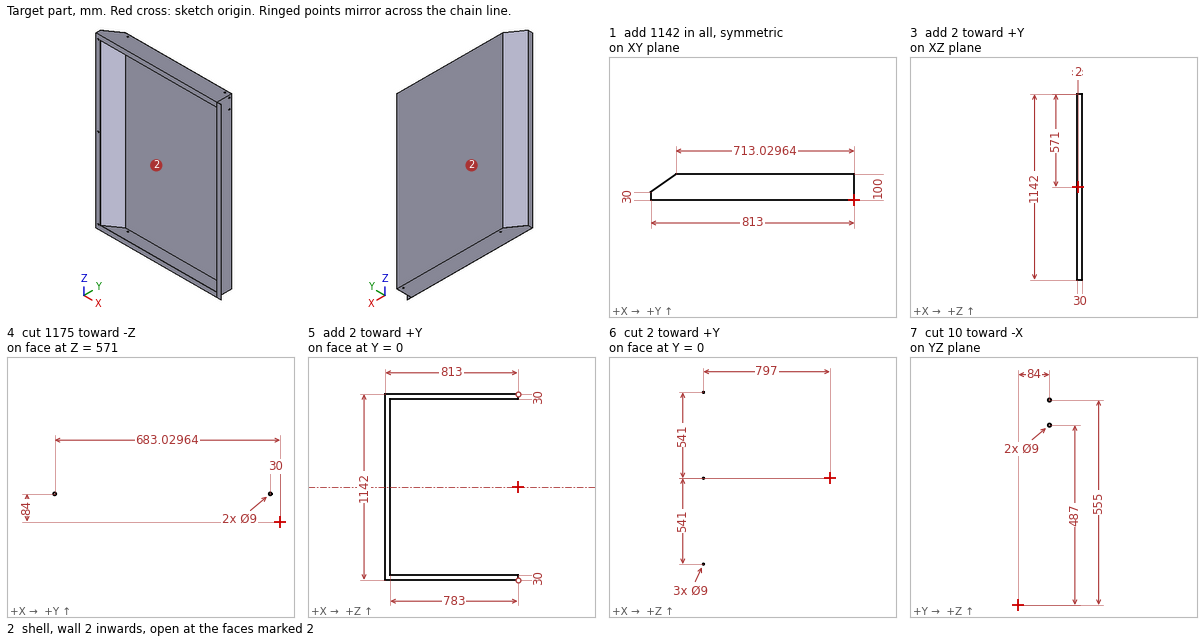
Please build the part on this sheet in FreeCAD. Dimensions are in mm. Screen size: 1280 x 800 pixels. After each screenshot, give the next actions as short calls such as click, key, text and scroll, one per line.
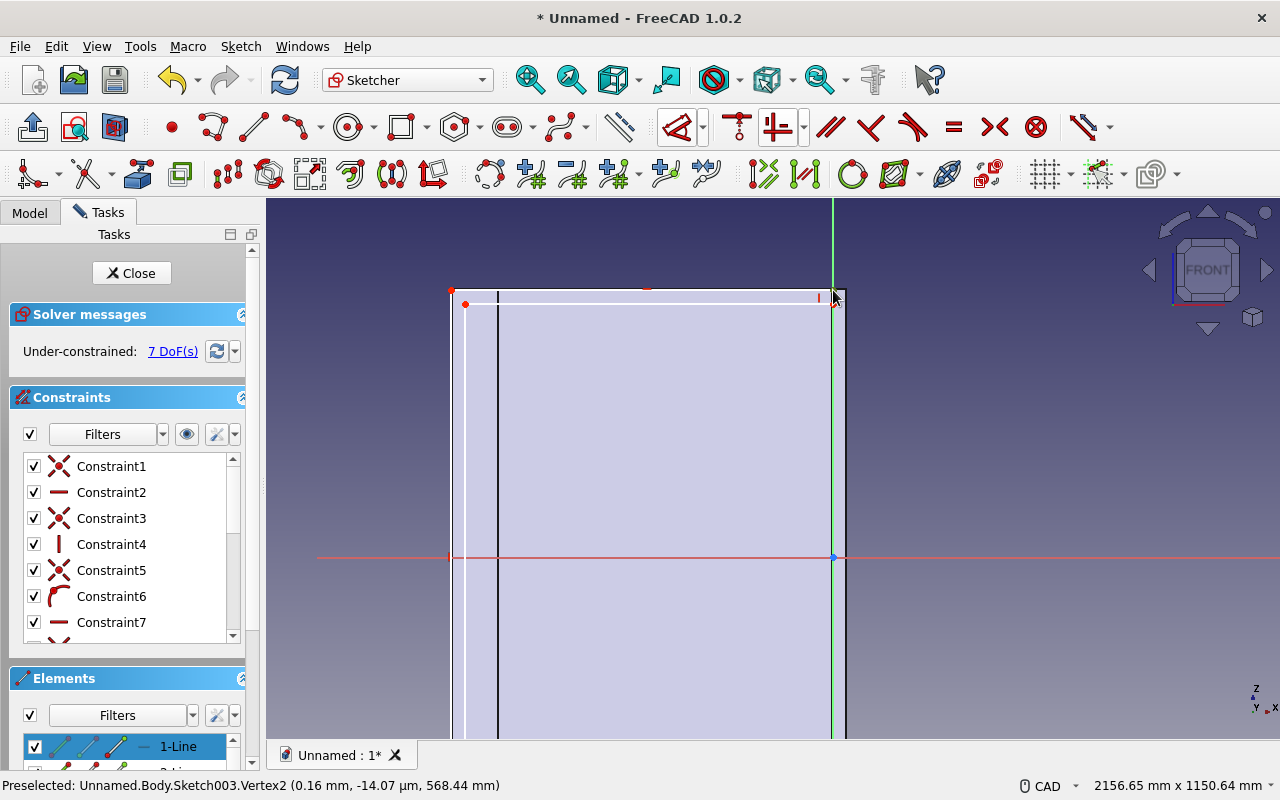
scroll(831, 288, down, 2)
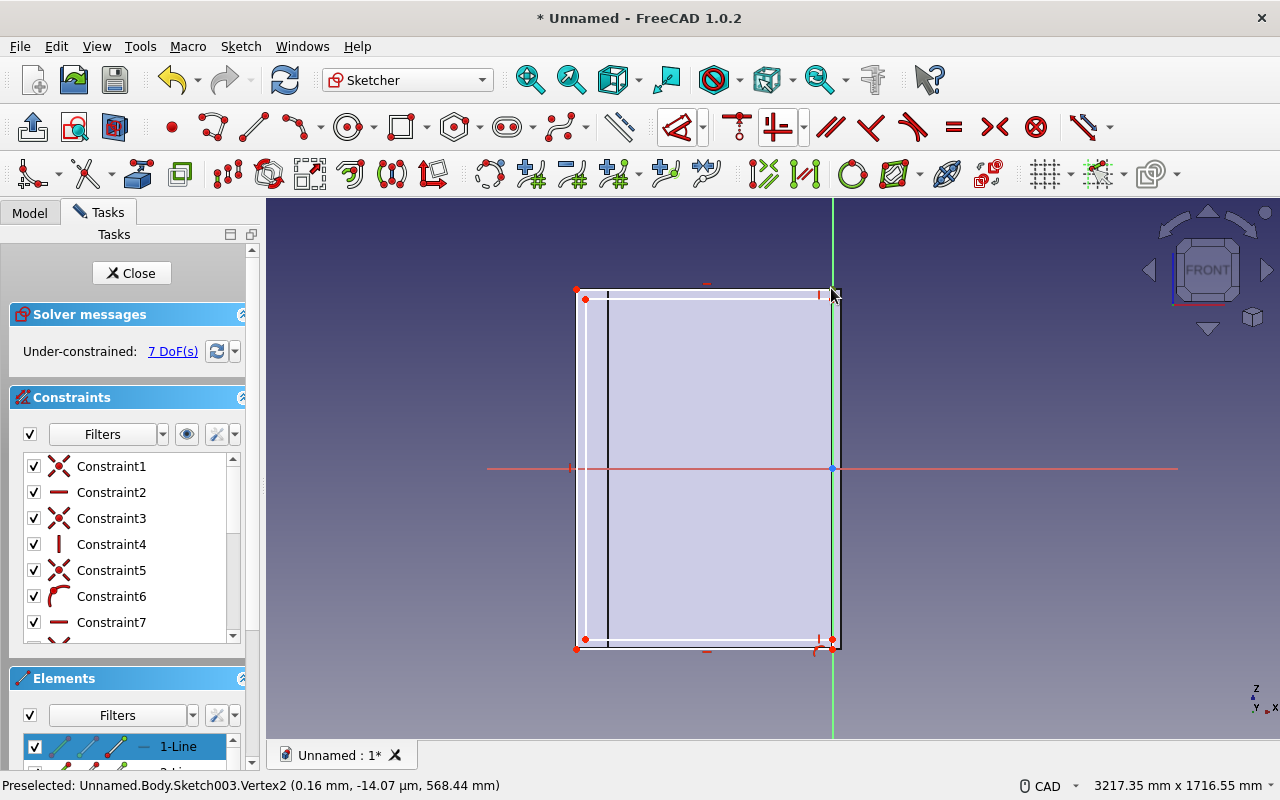
scroll(833, 649, up, 2)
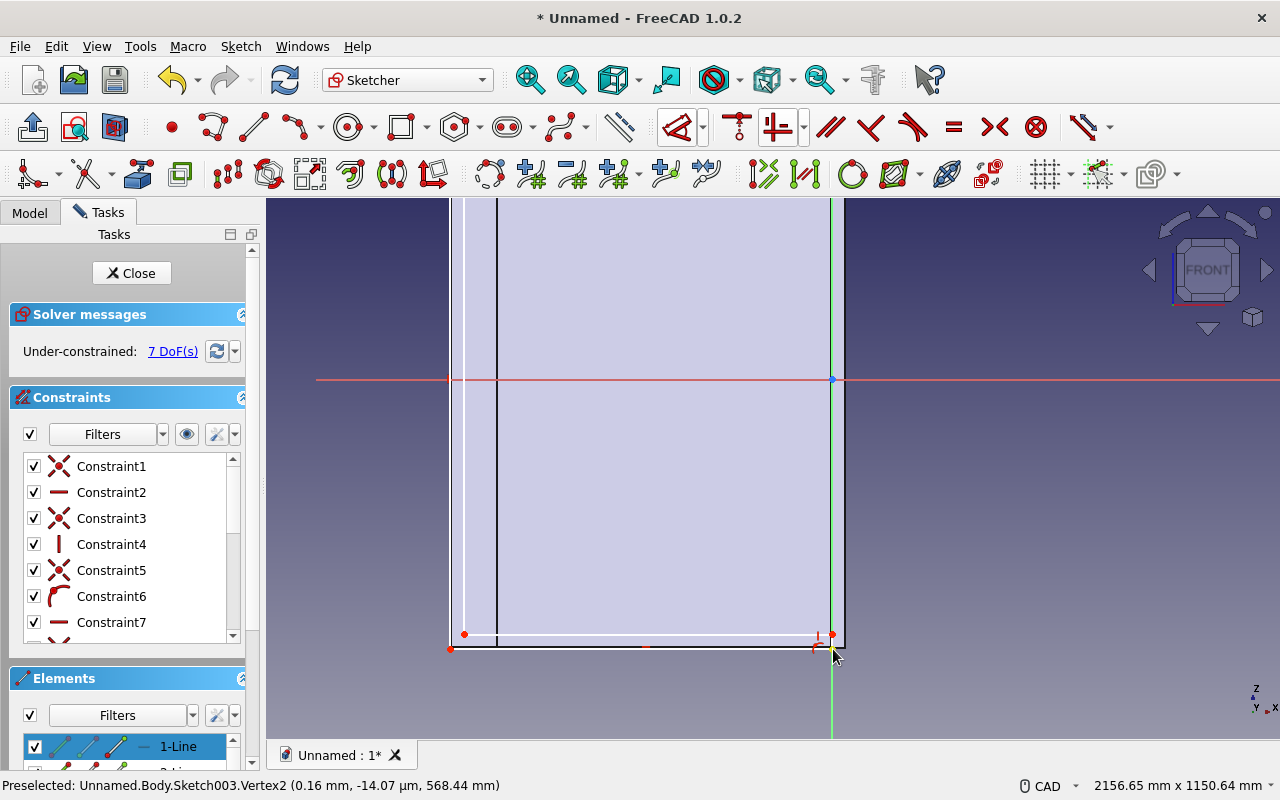
click(832, 649)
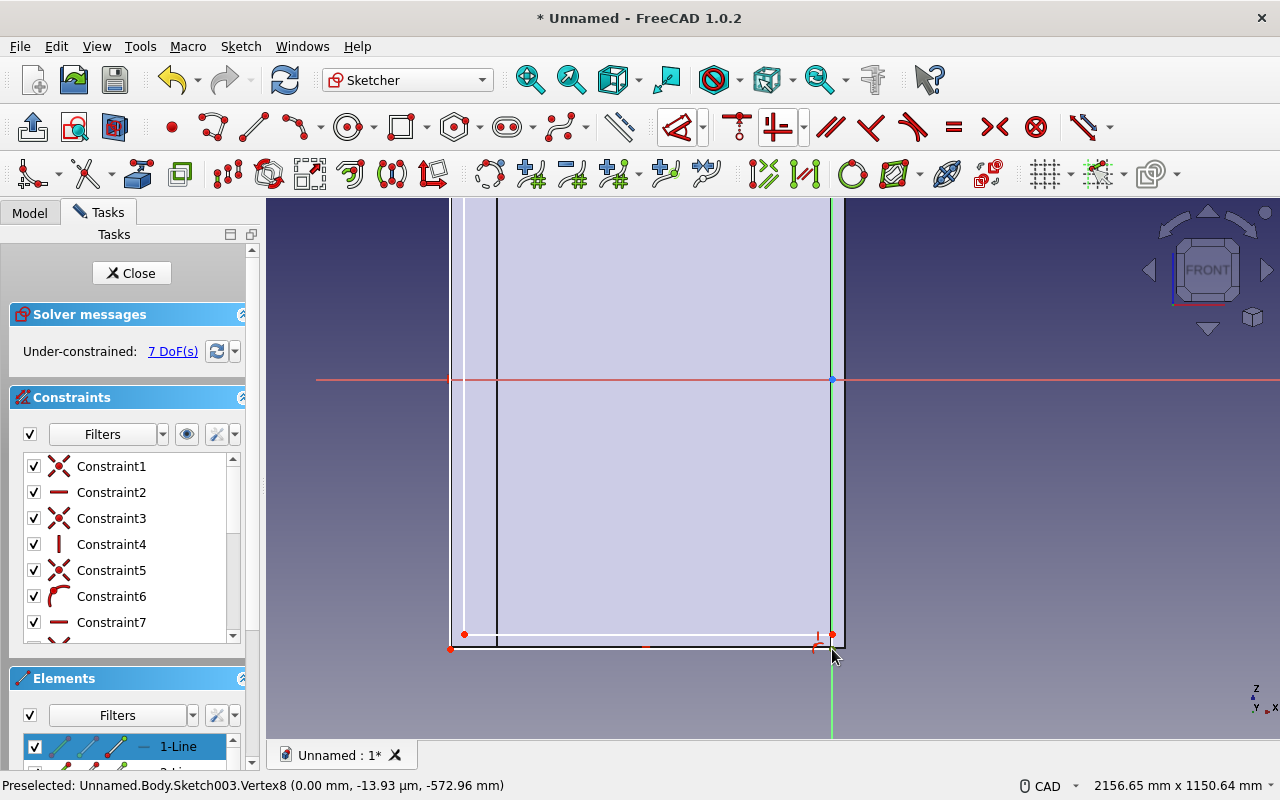
click(353, 380)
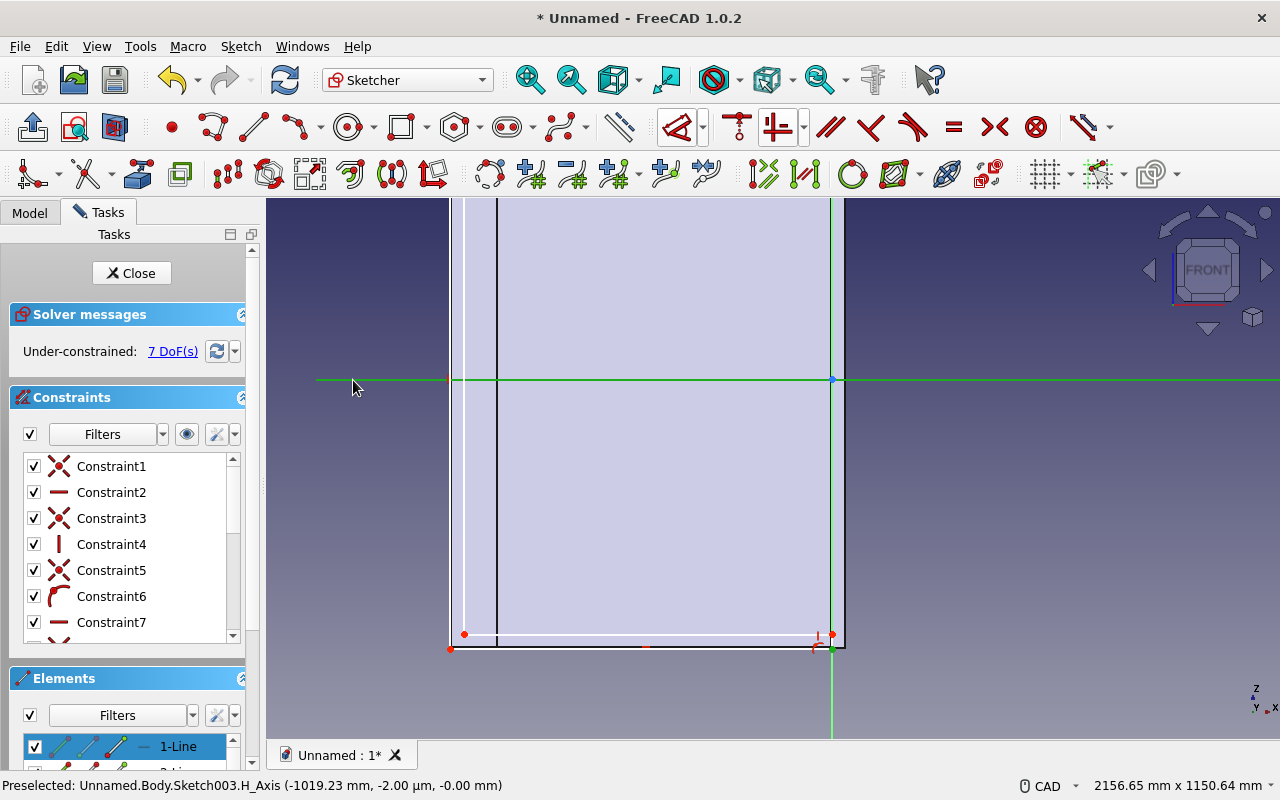
click(995, 128)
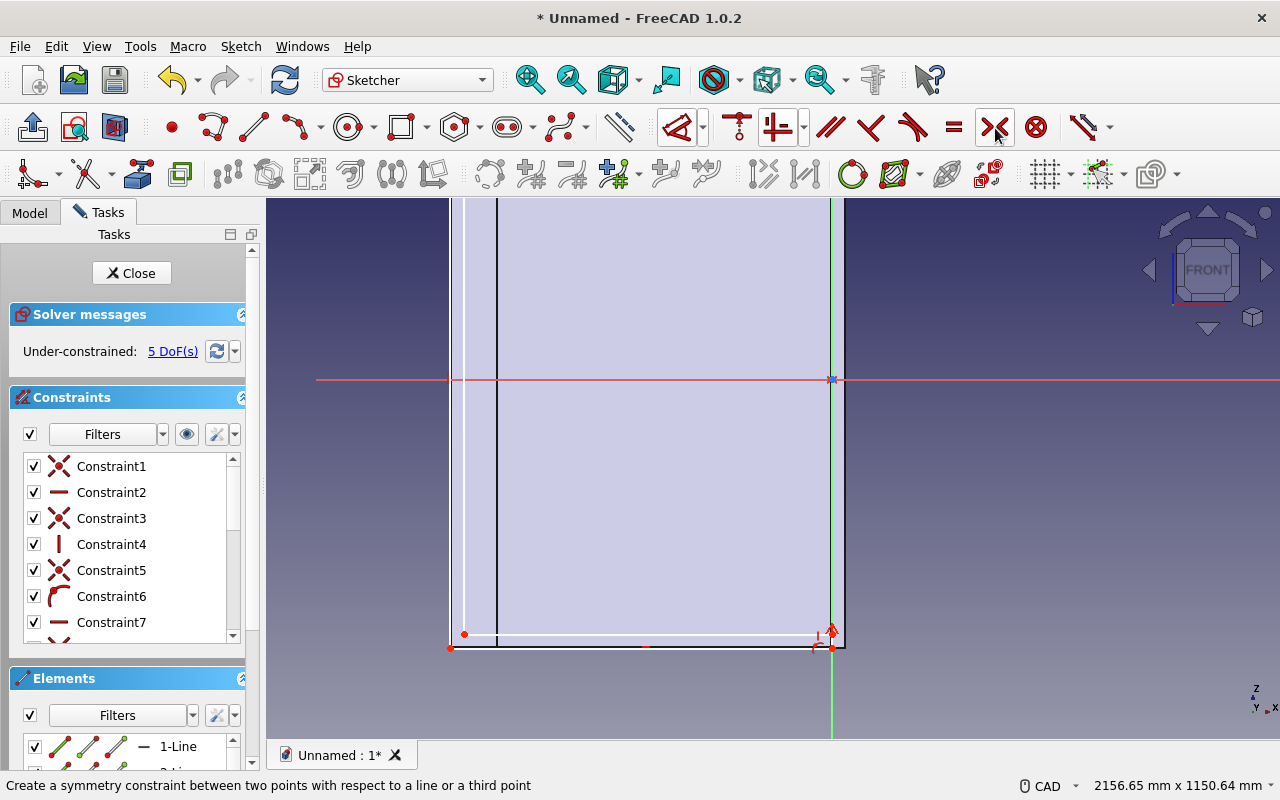
scroll(833, 649, down, 2)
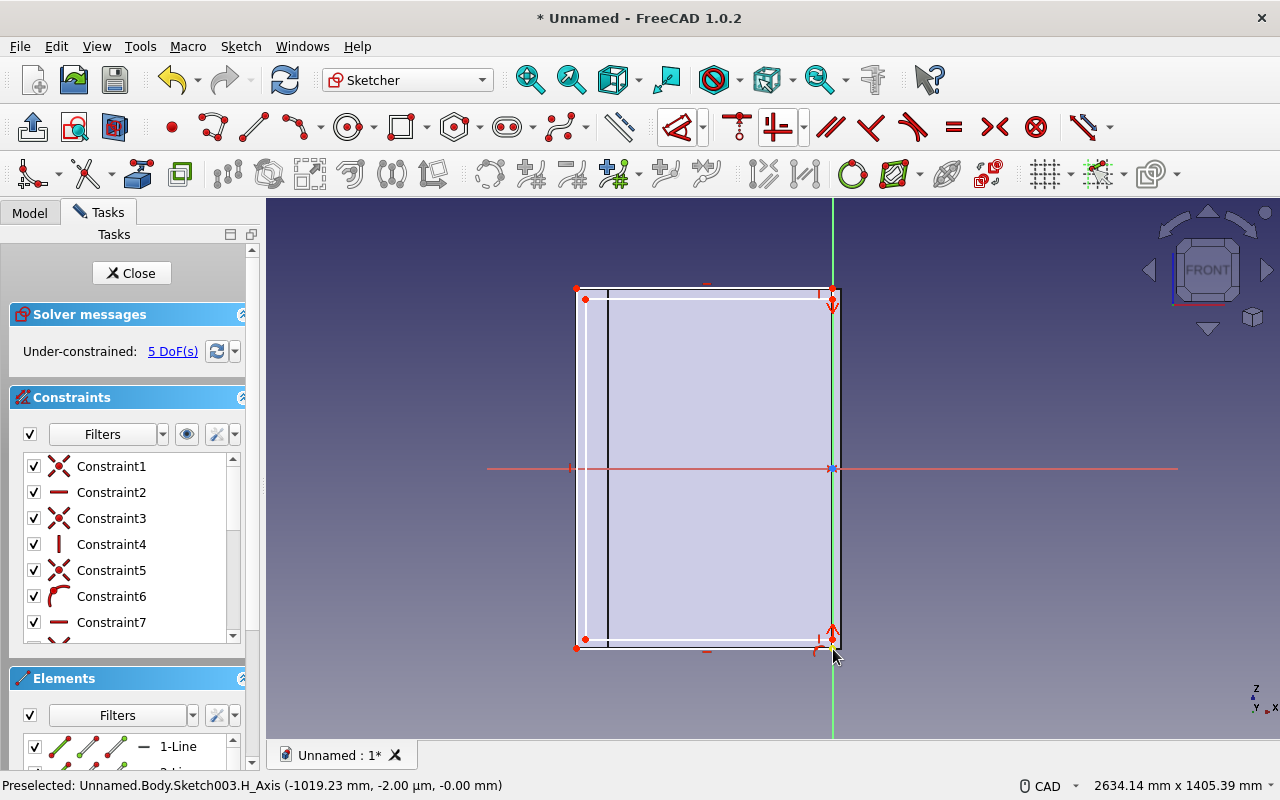
scroll(833, 294, up, 8)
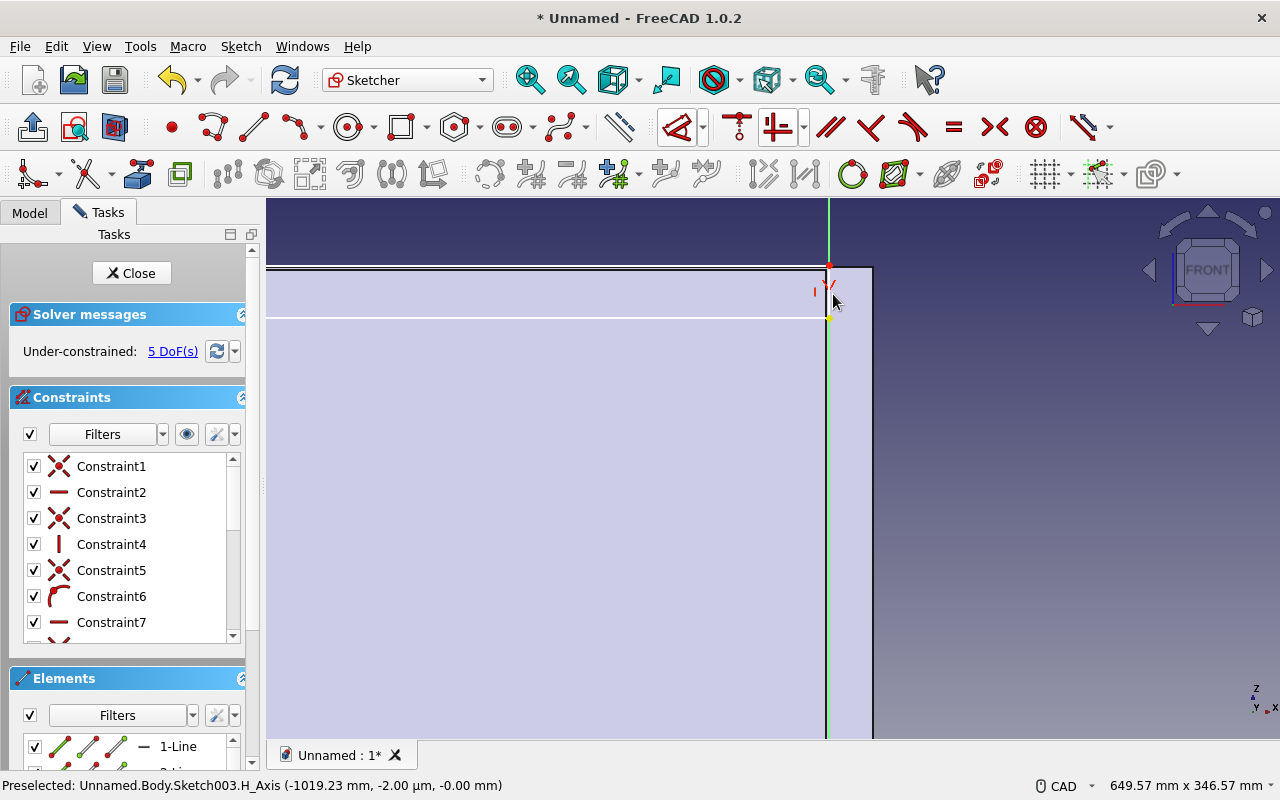
click(829, 297)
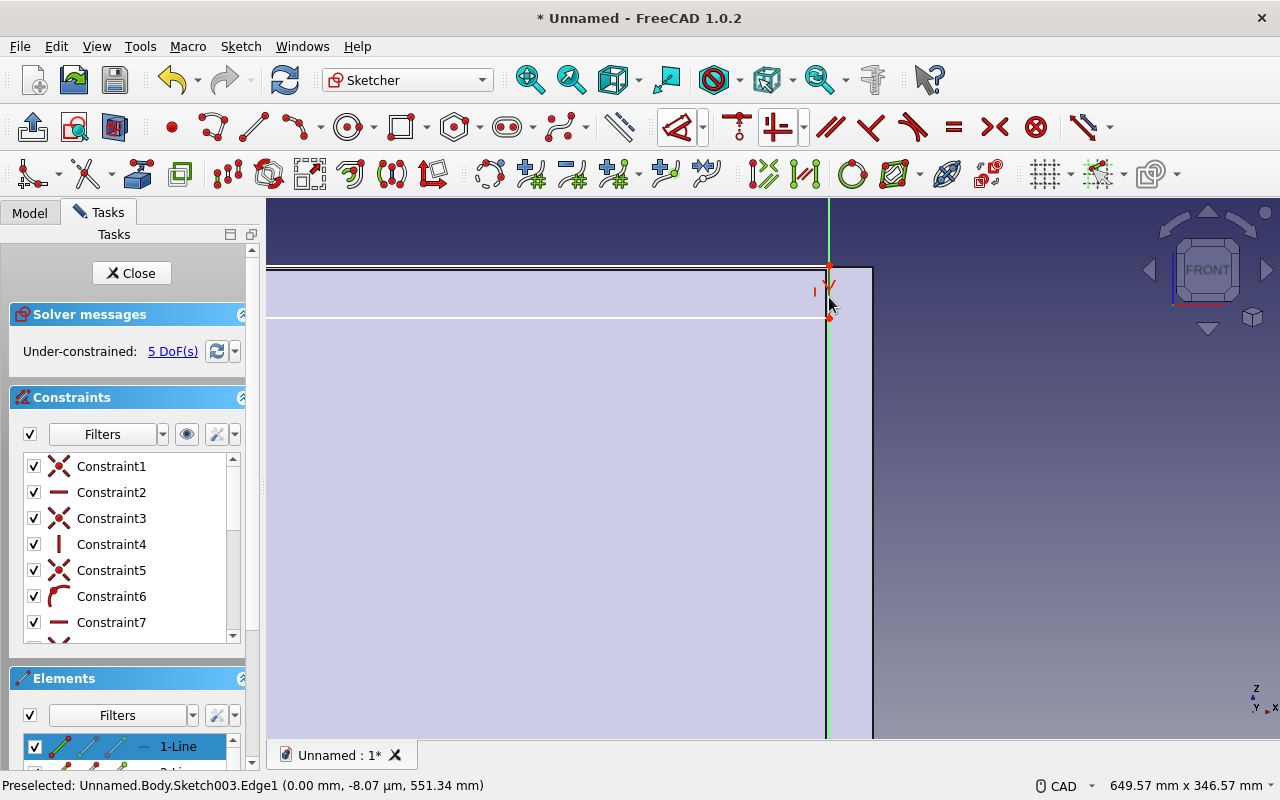
key(i)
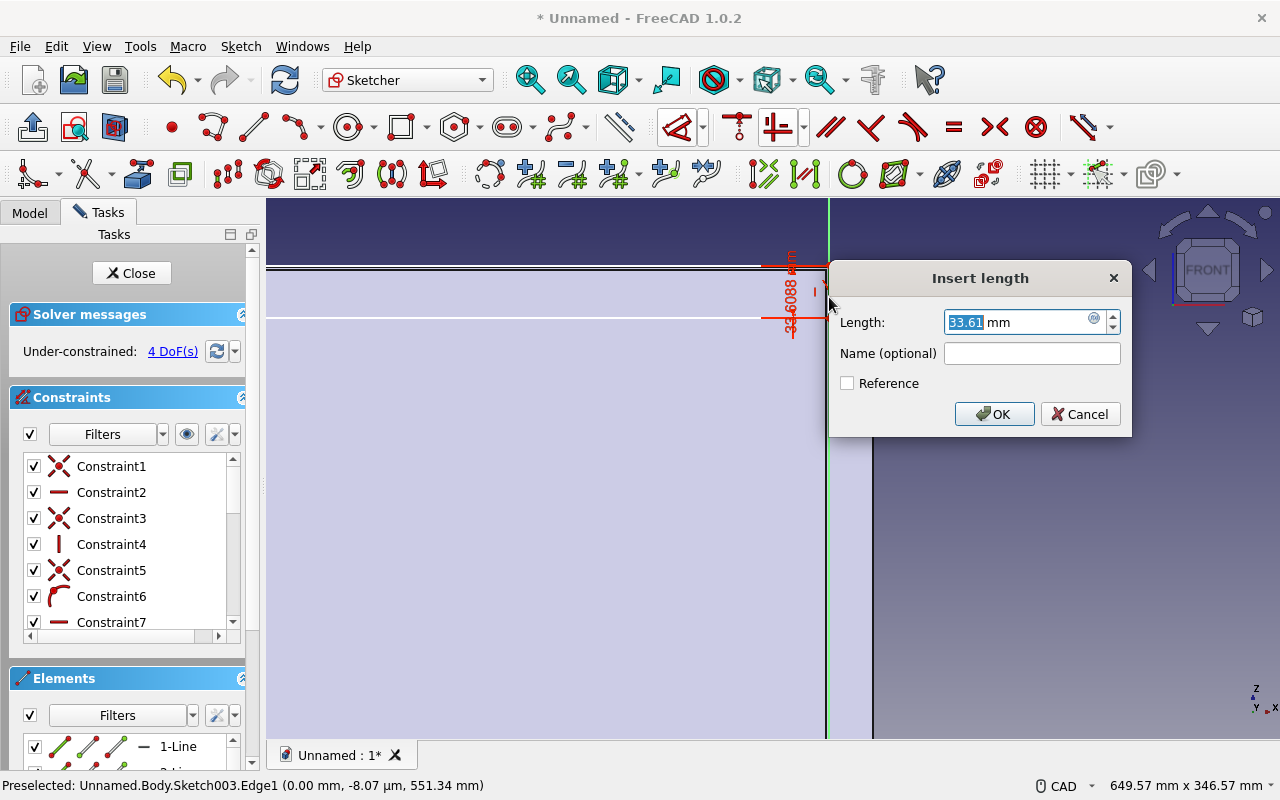
text(30)
key(Return)